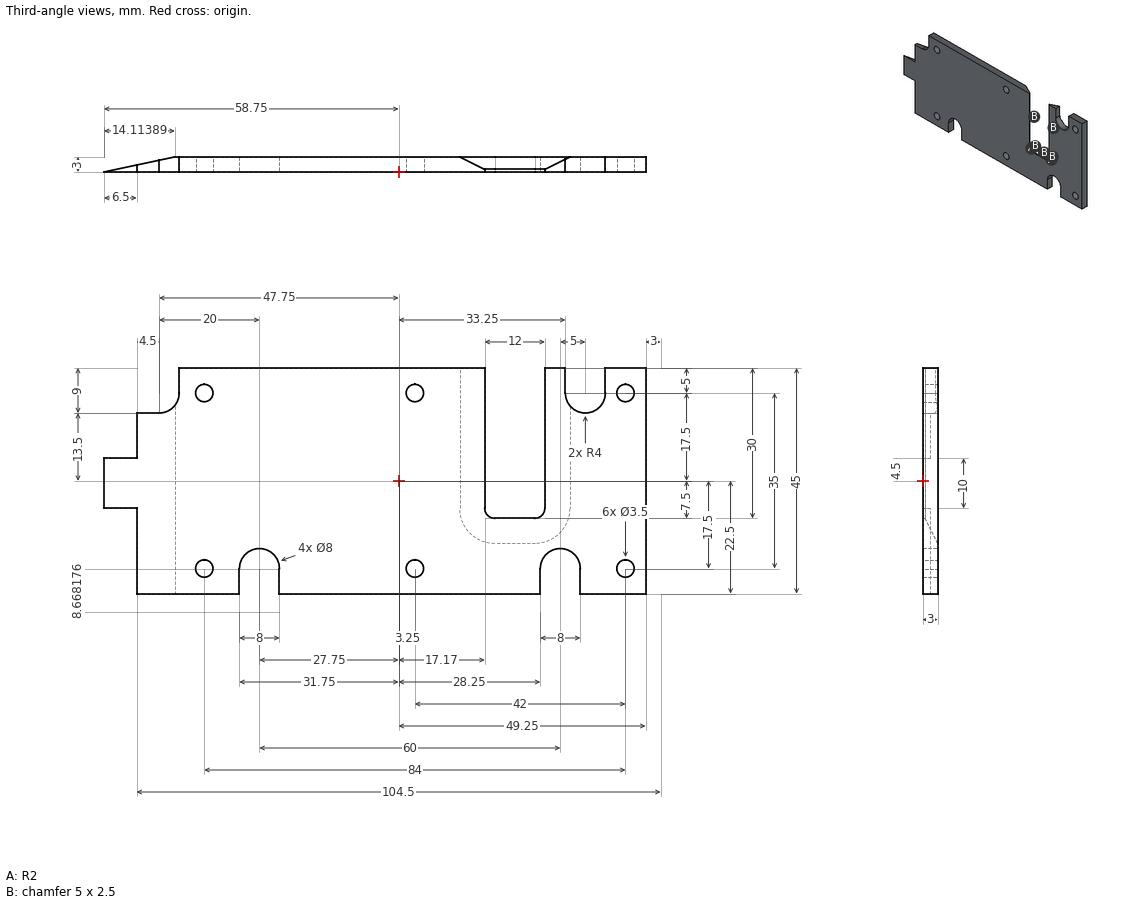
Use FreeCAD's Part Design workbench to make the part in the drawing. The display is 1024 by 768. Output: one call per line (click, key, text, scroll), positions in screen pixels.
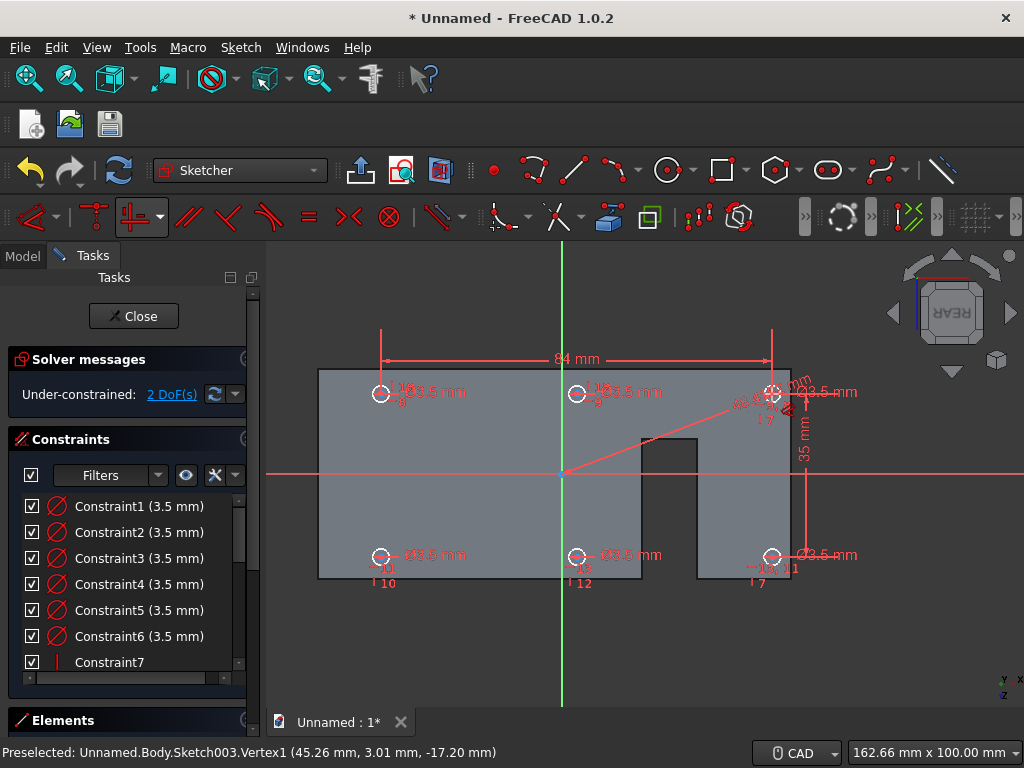
click(577, 394)
click(675, 360)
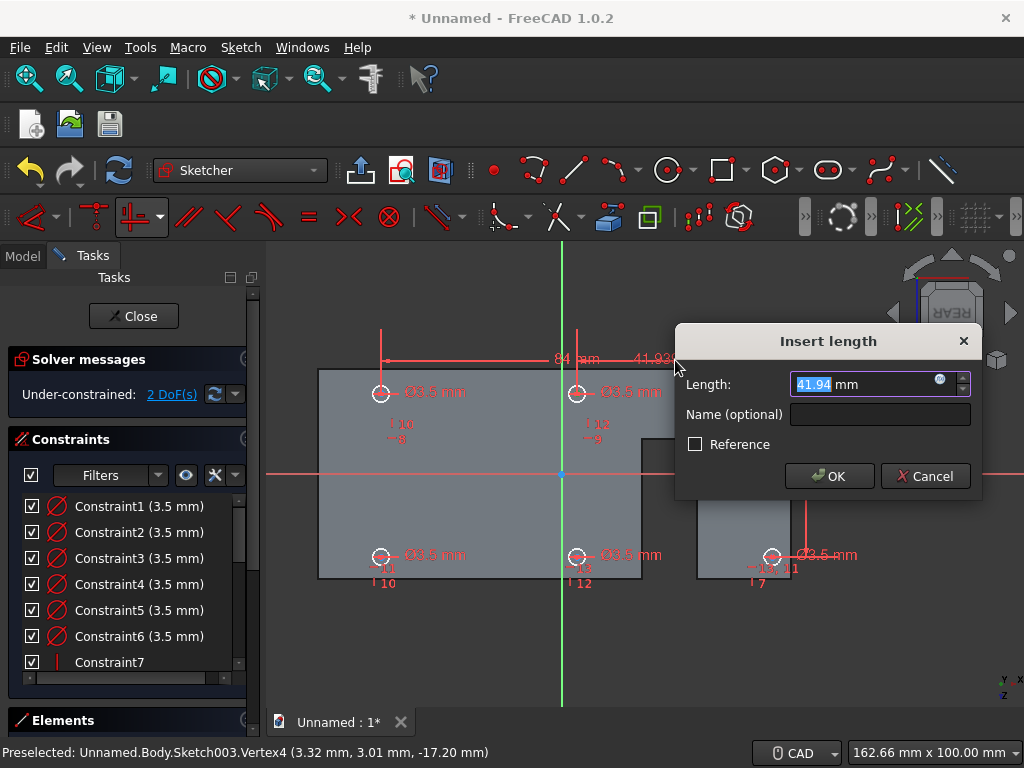
text(42)
key(Return)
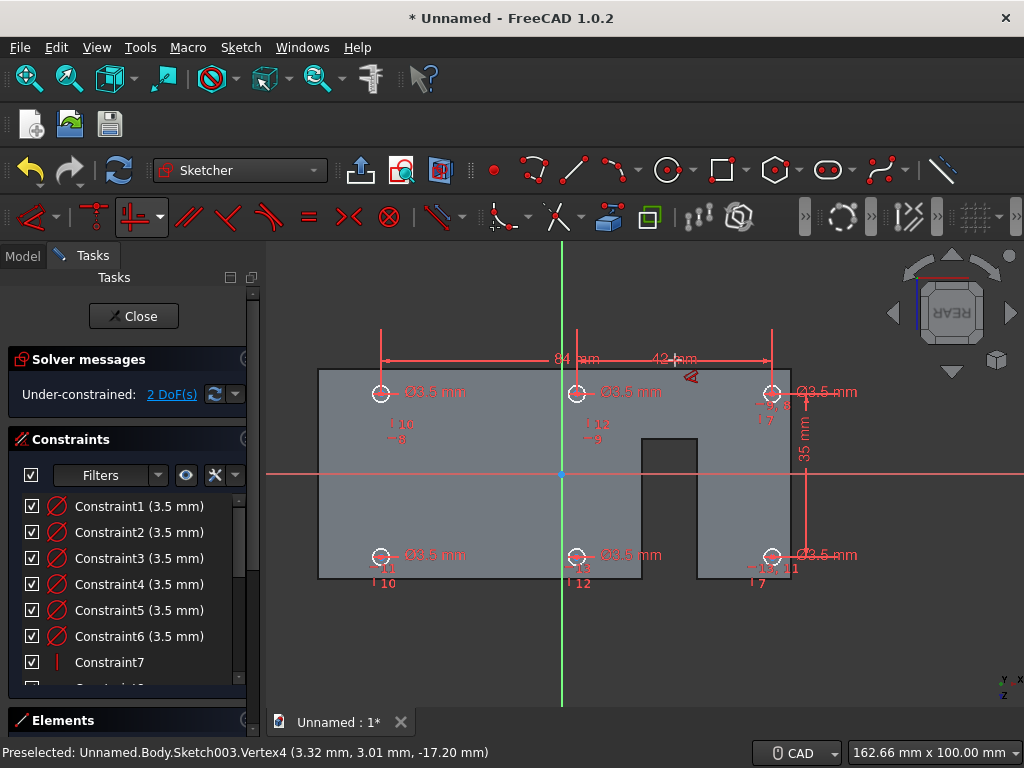
click(772, 394)
click(806, 416)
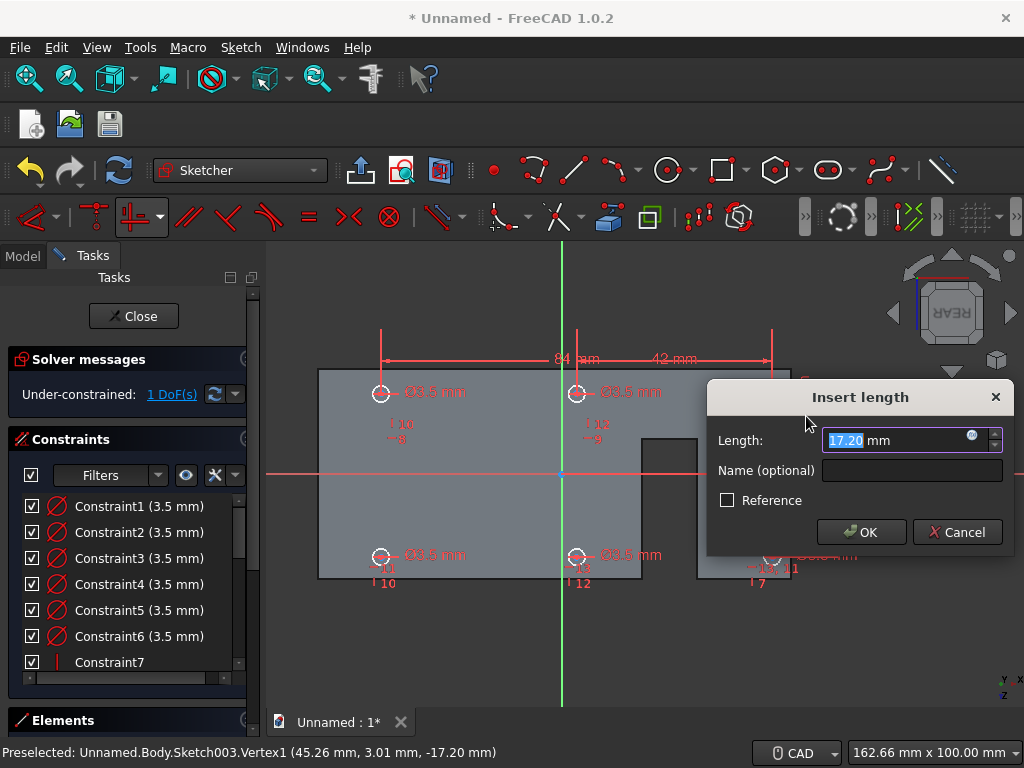
text(17.5)
key(Return)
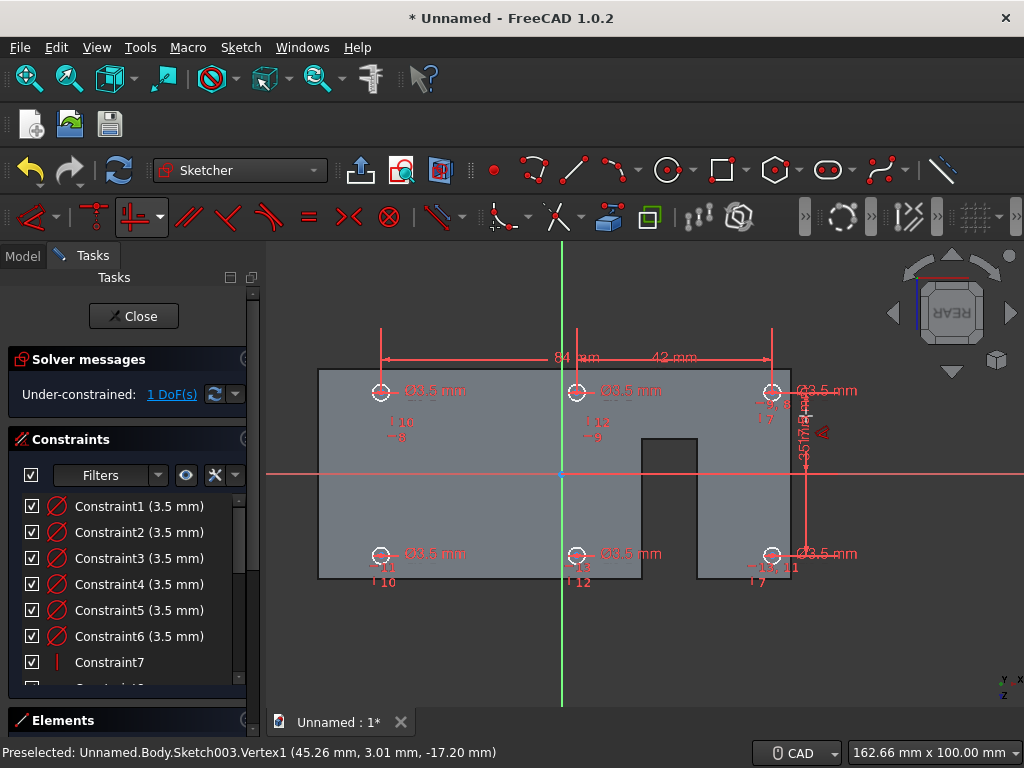
scroll(577, 393, up, 5)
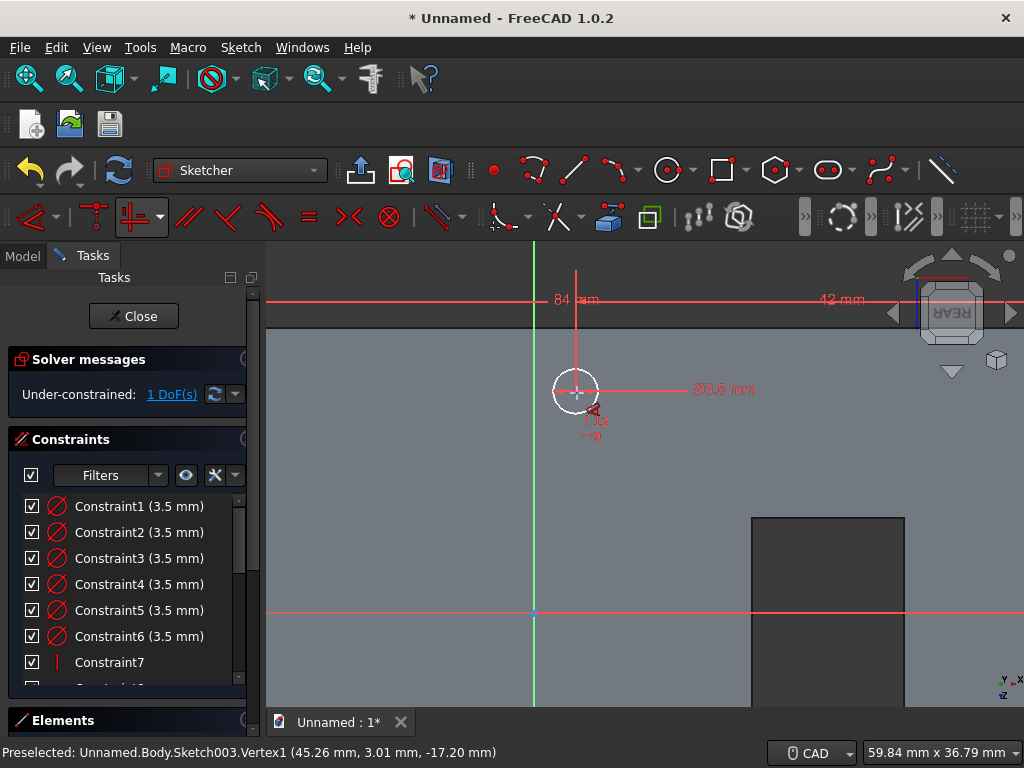
click(576, 391)
click(555, 357)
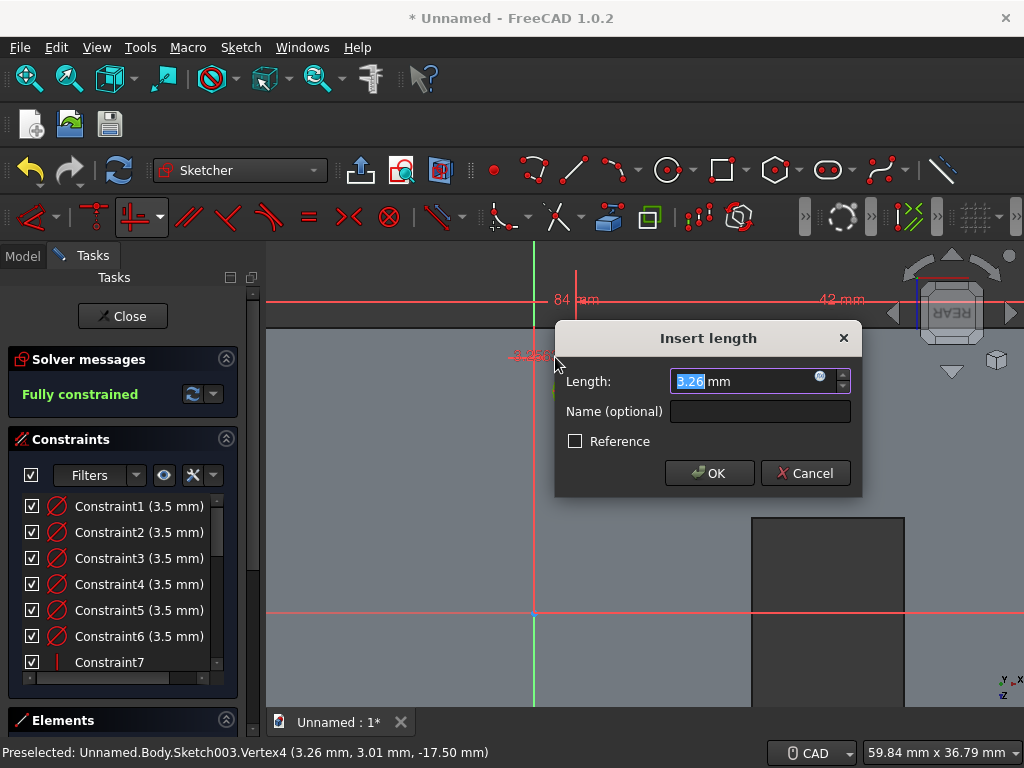
text(3.25)
key(Return)
key(Escape)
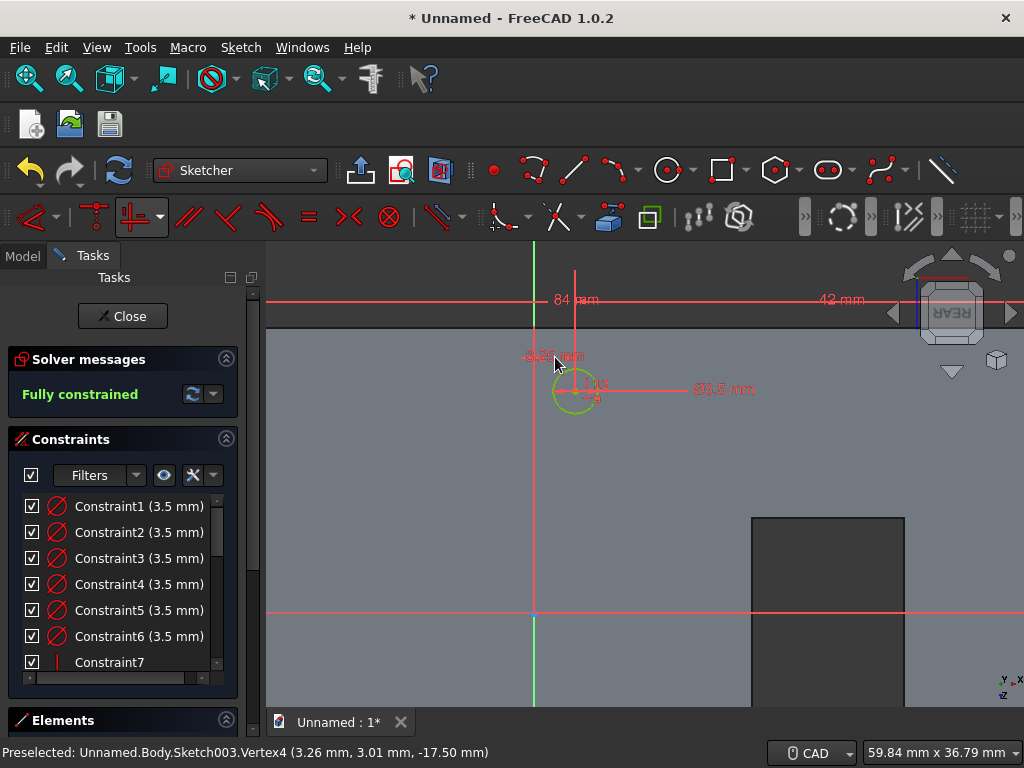
click(123, 316)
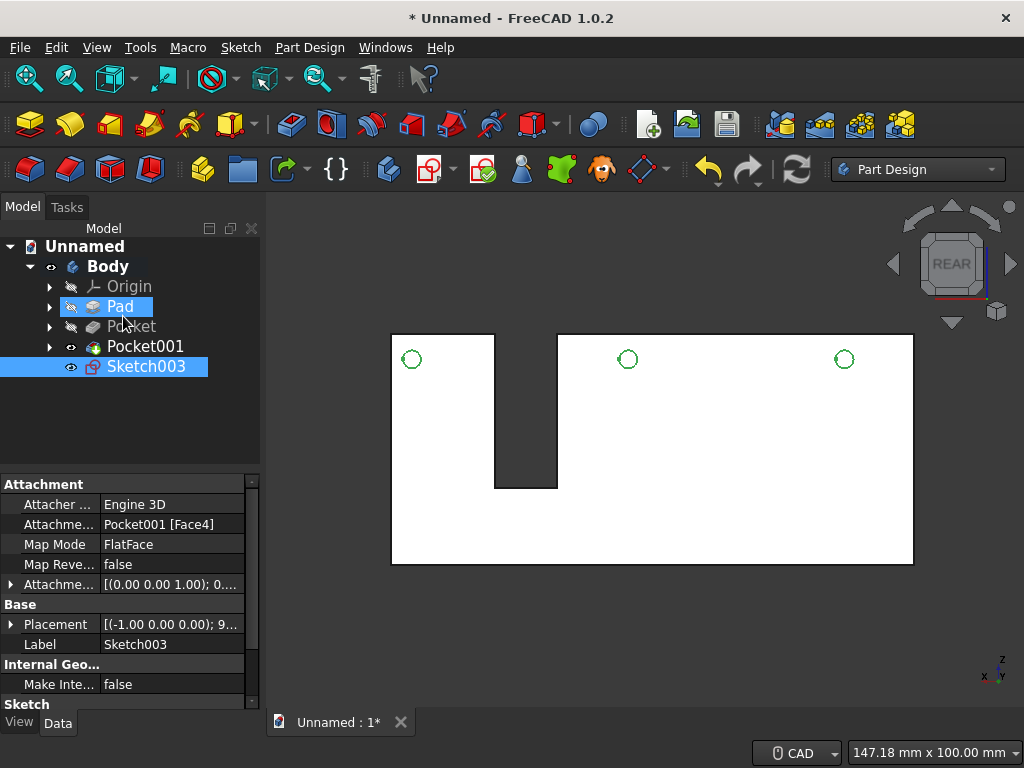
click(292, 124)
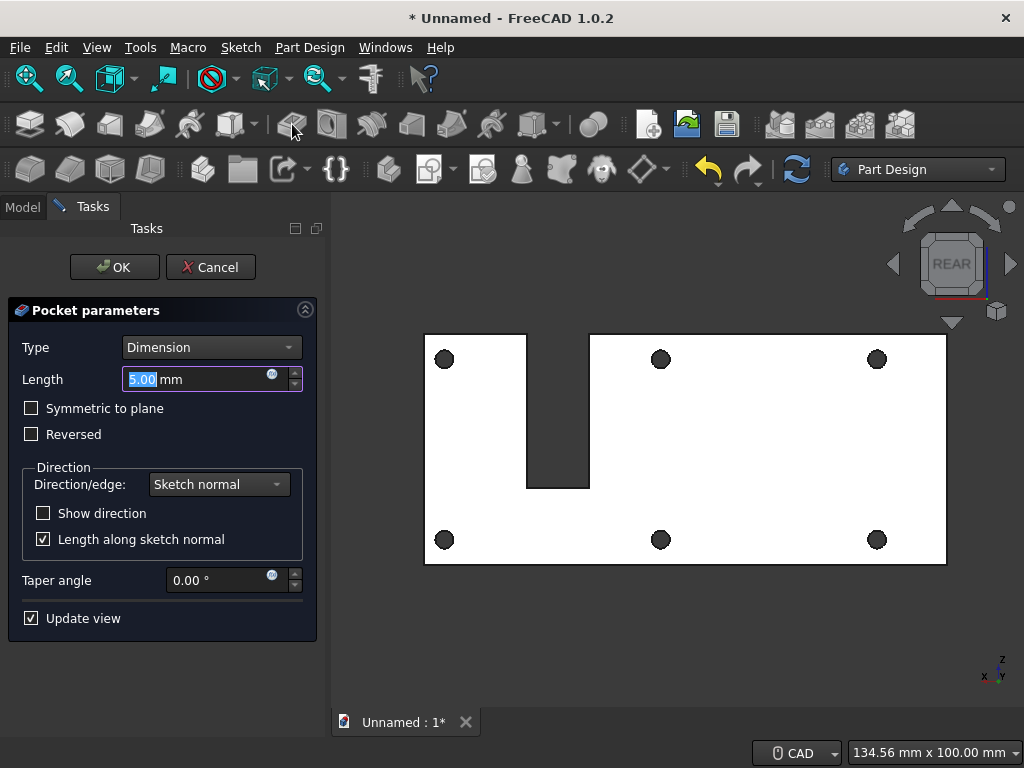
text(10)
key(Tab)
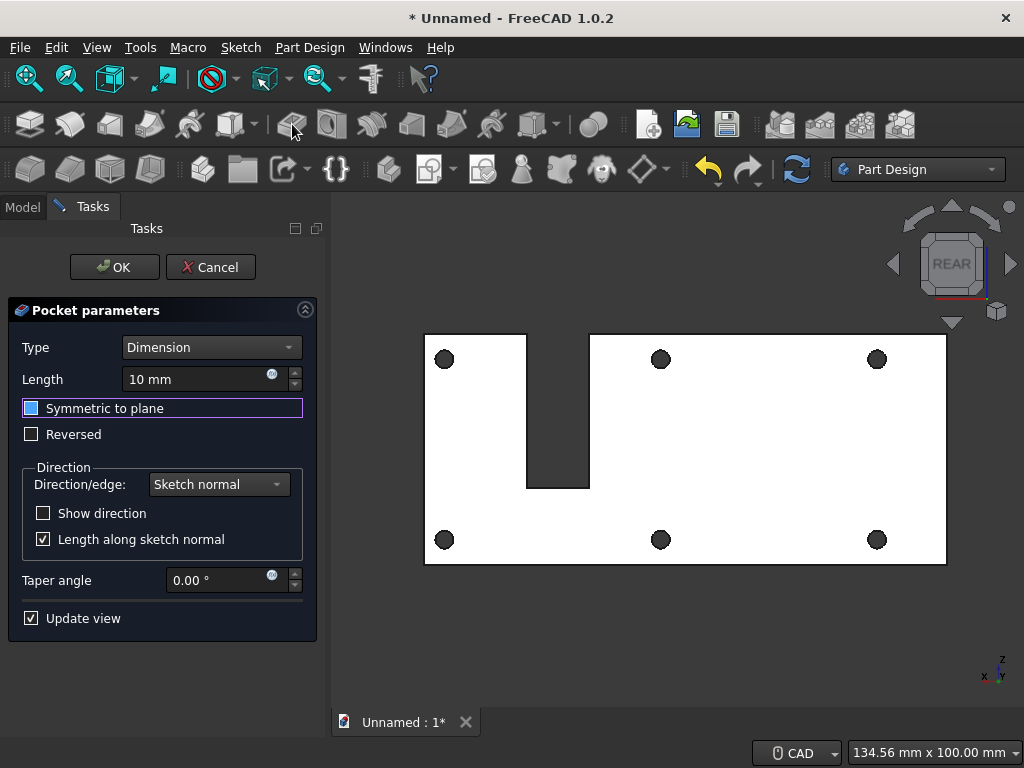
click(115, 267)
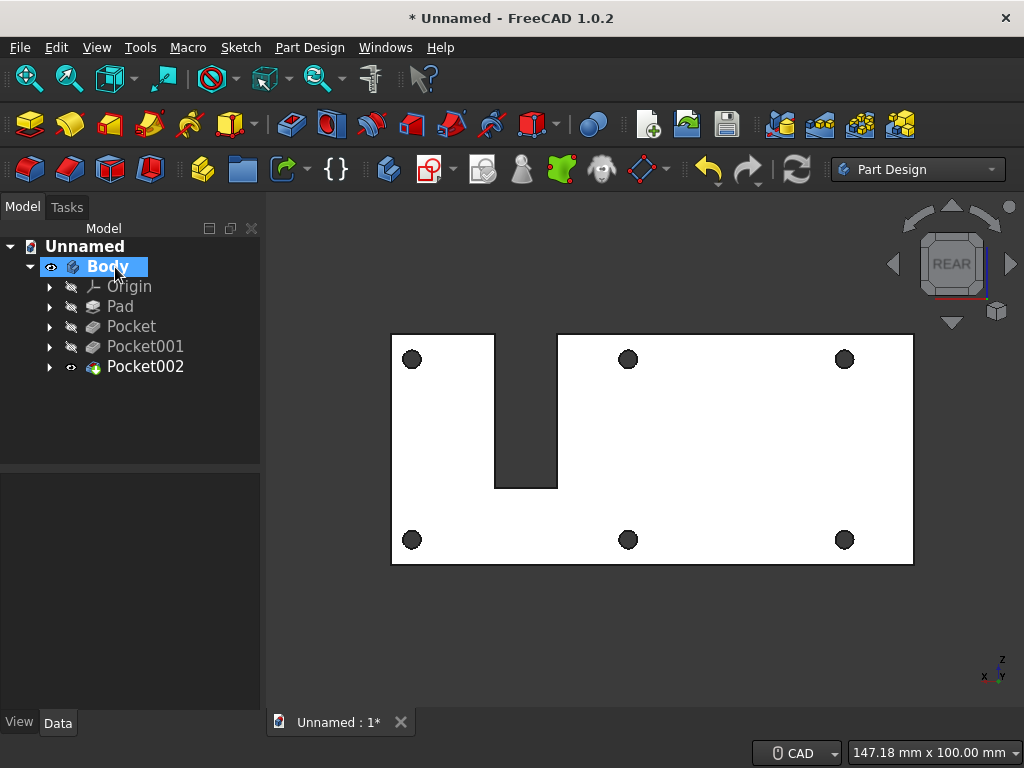
key(6)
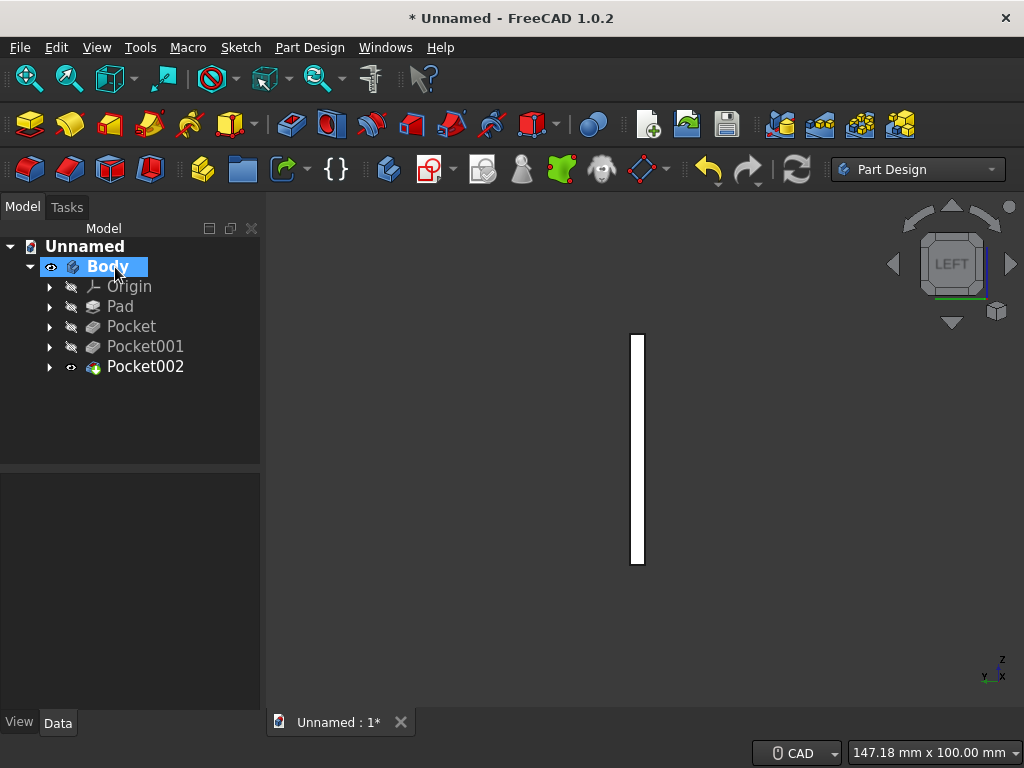
key(v)
key(f)